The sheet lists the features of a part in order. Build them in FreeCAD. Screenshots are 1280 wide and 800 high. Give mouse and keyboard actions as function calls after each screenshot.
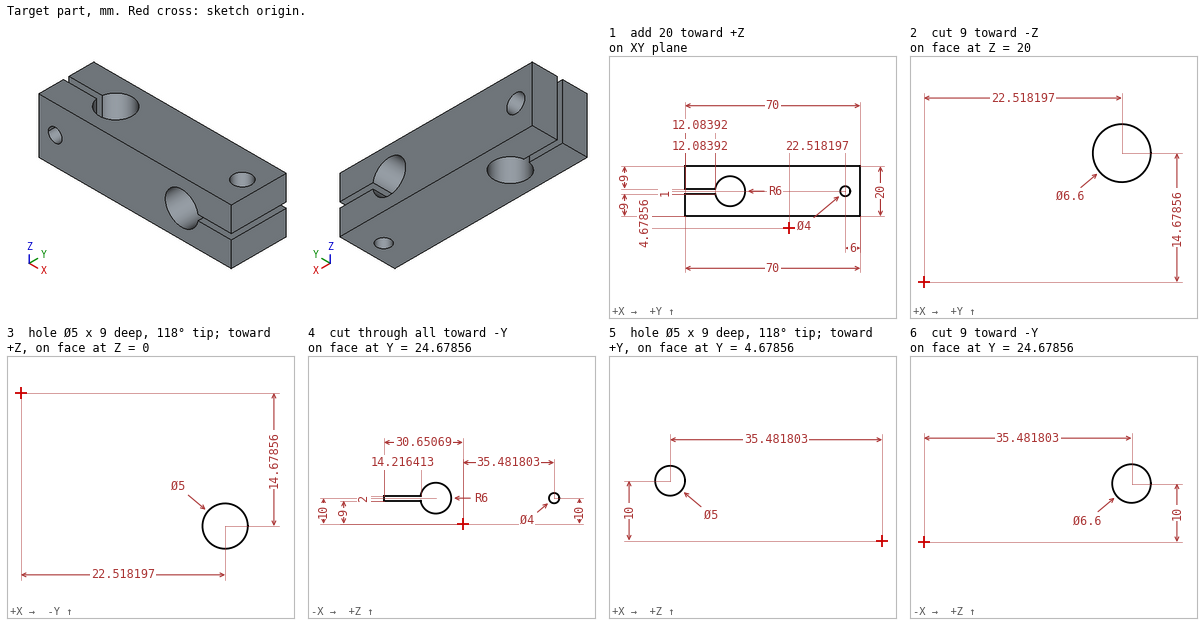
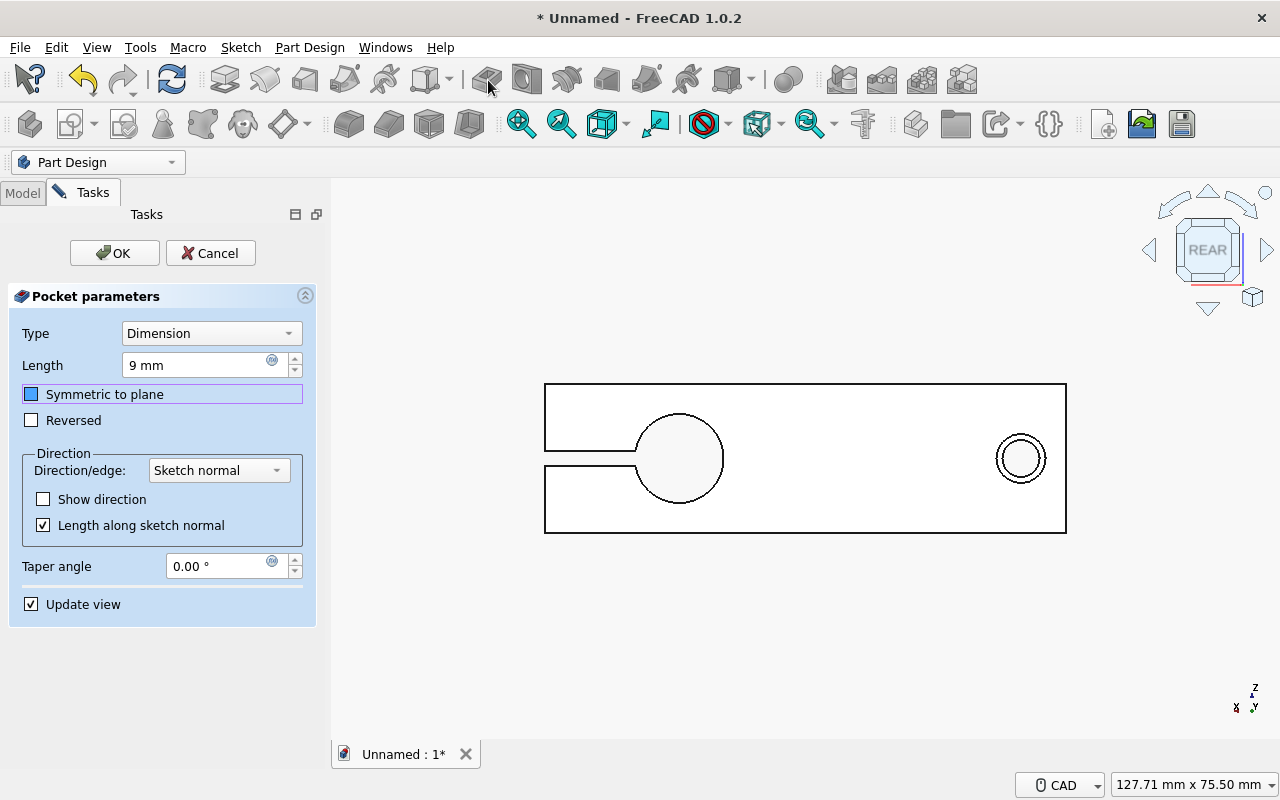
click(115, 253)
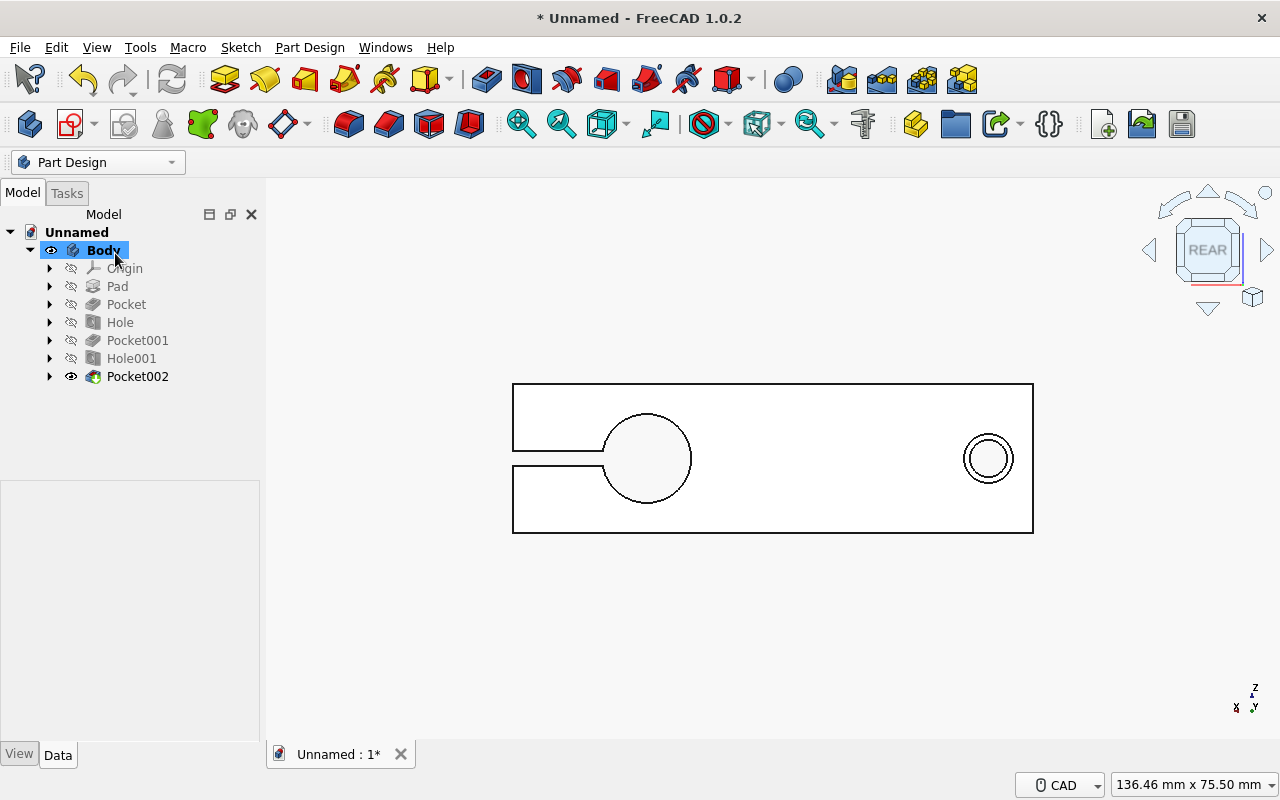
key(0)